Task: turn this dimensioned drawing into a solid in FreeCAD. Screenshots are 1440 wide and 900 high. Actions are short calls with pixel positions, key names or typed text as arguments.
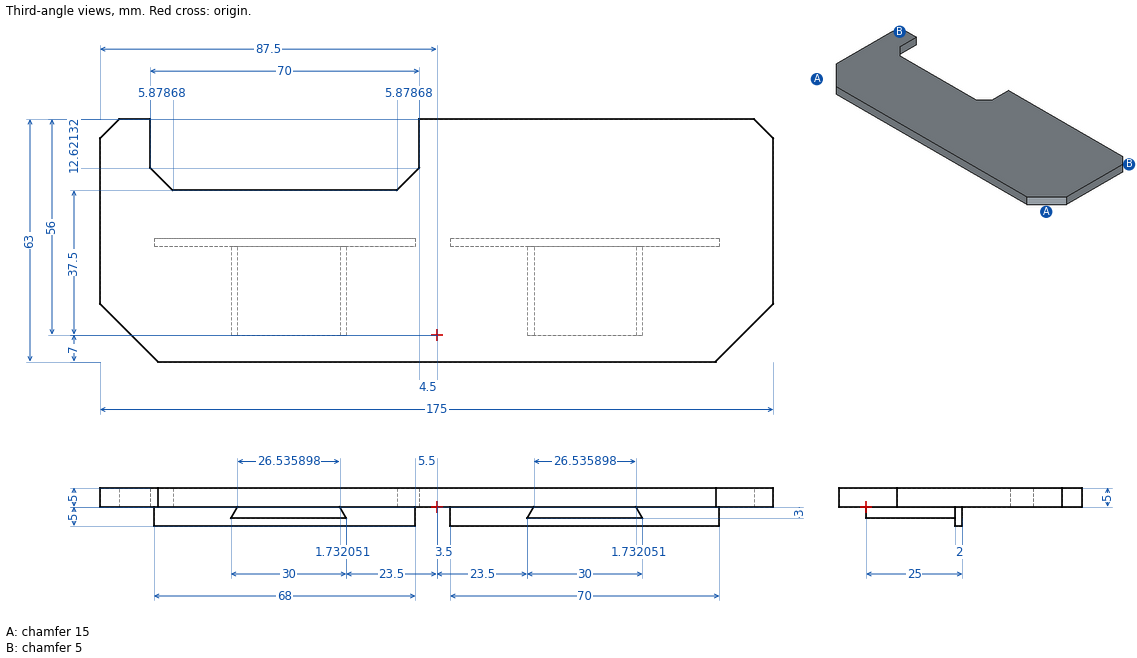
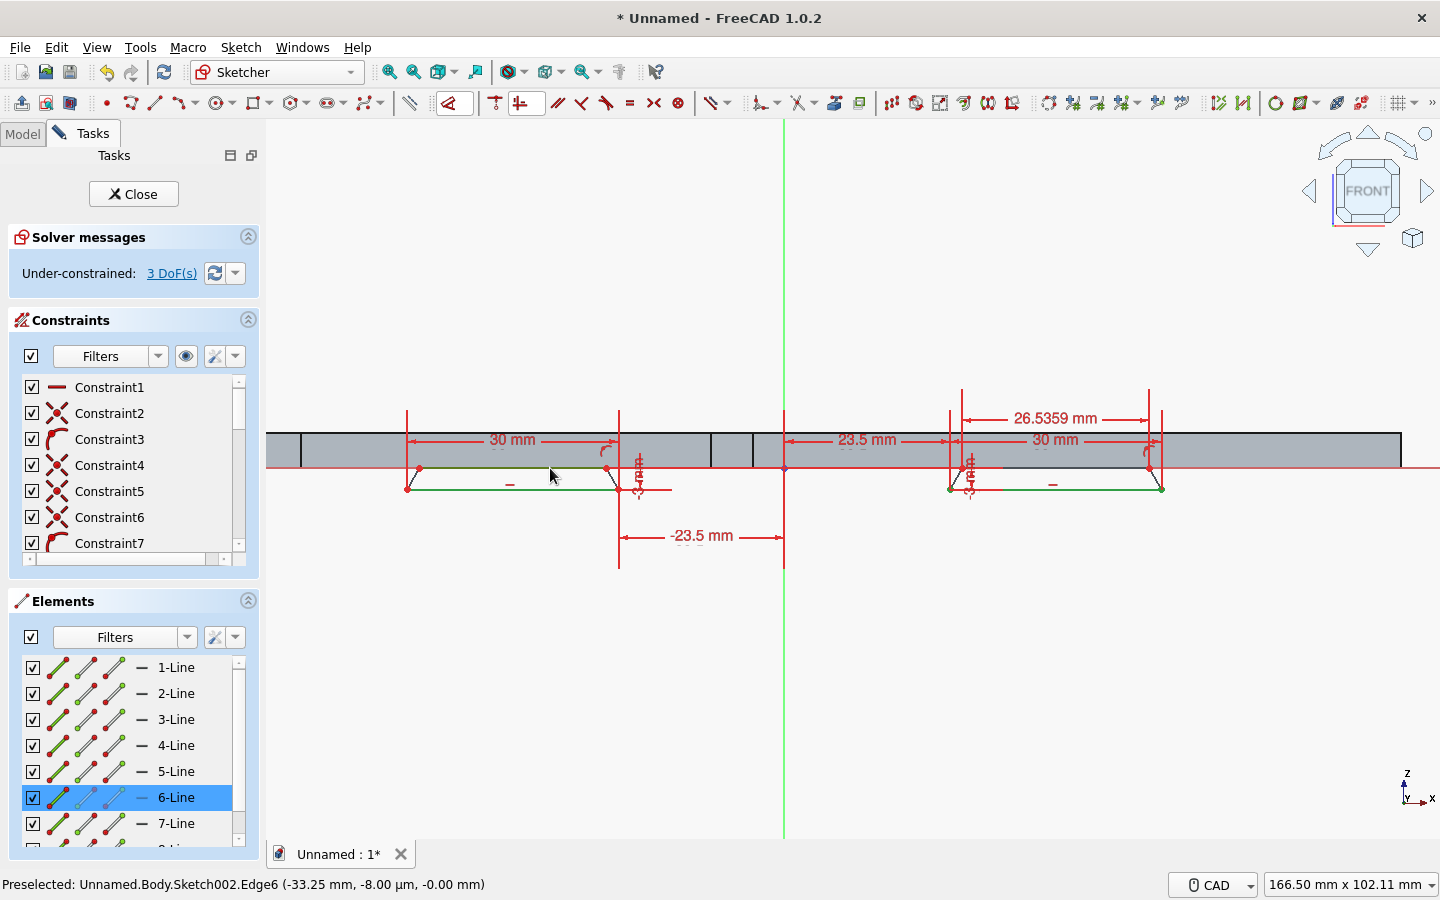
key(l)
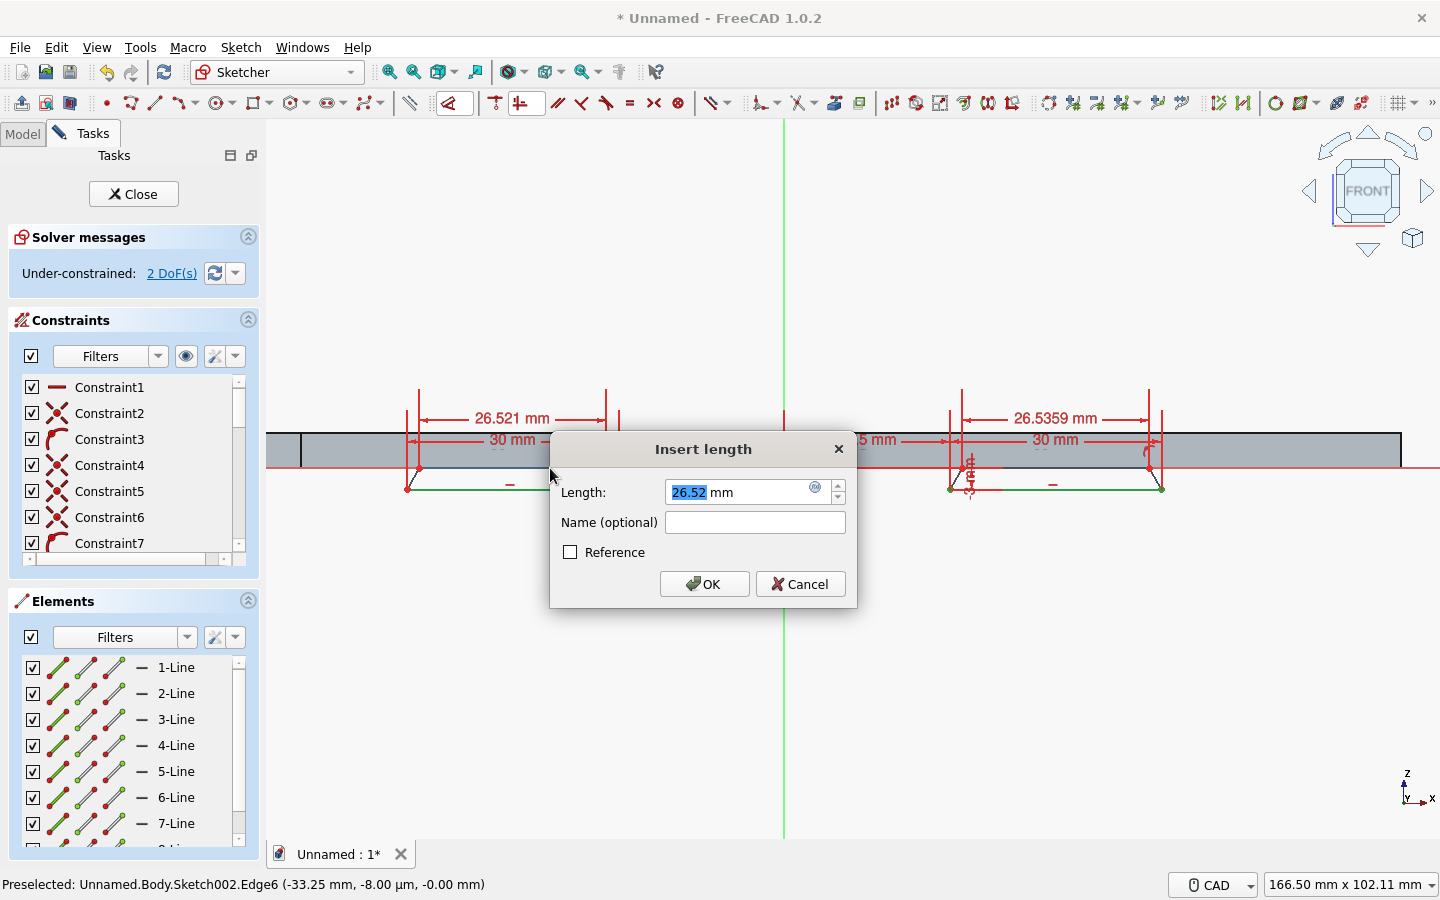
text(26.535898)
key(Return)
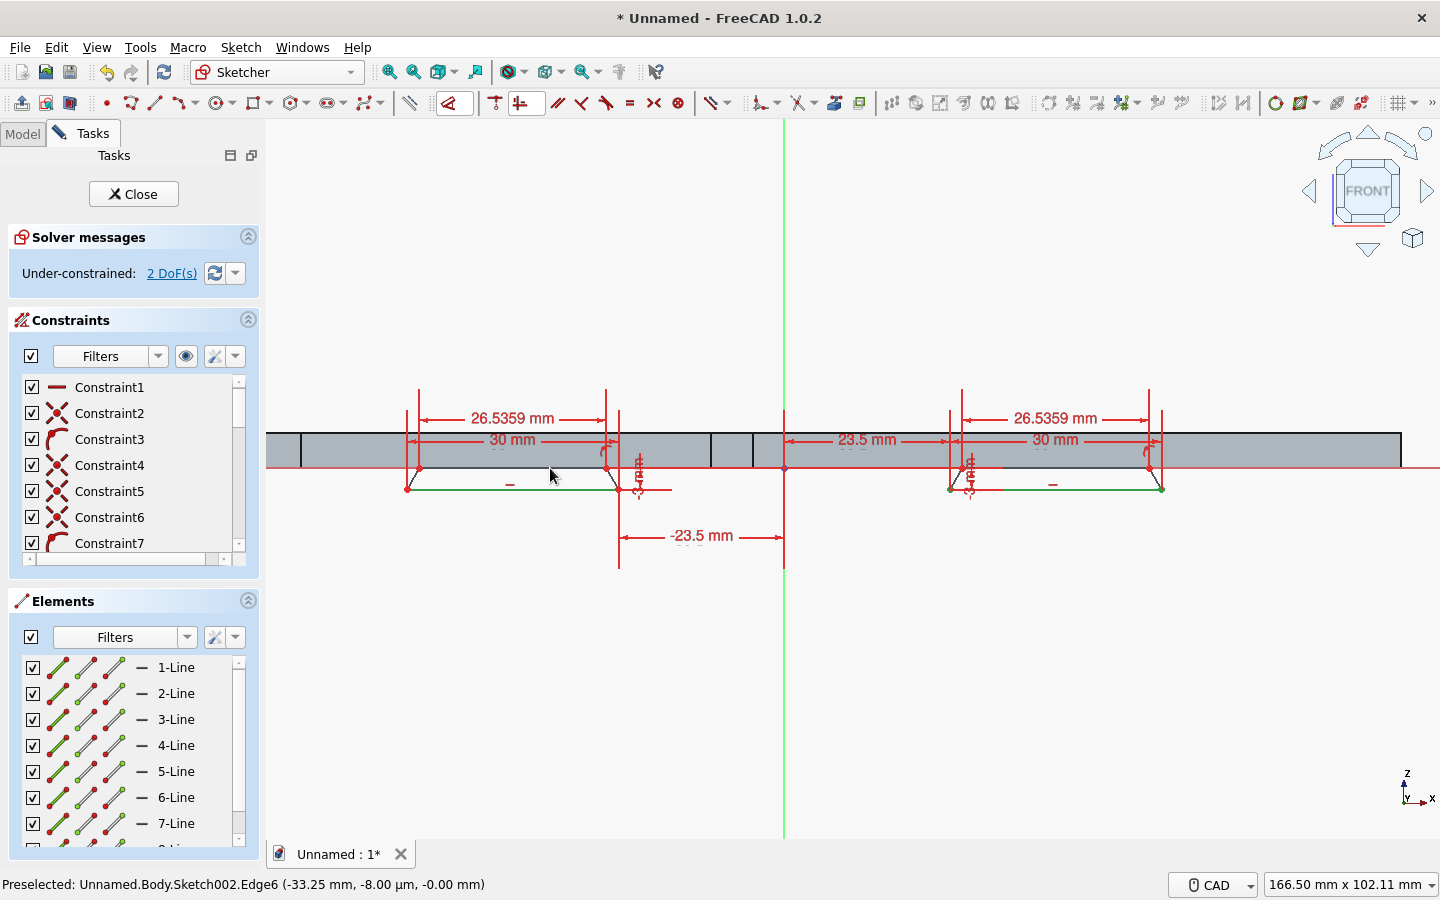
scroll(1155, 479, up, 6)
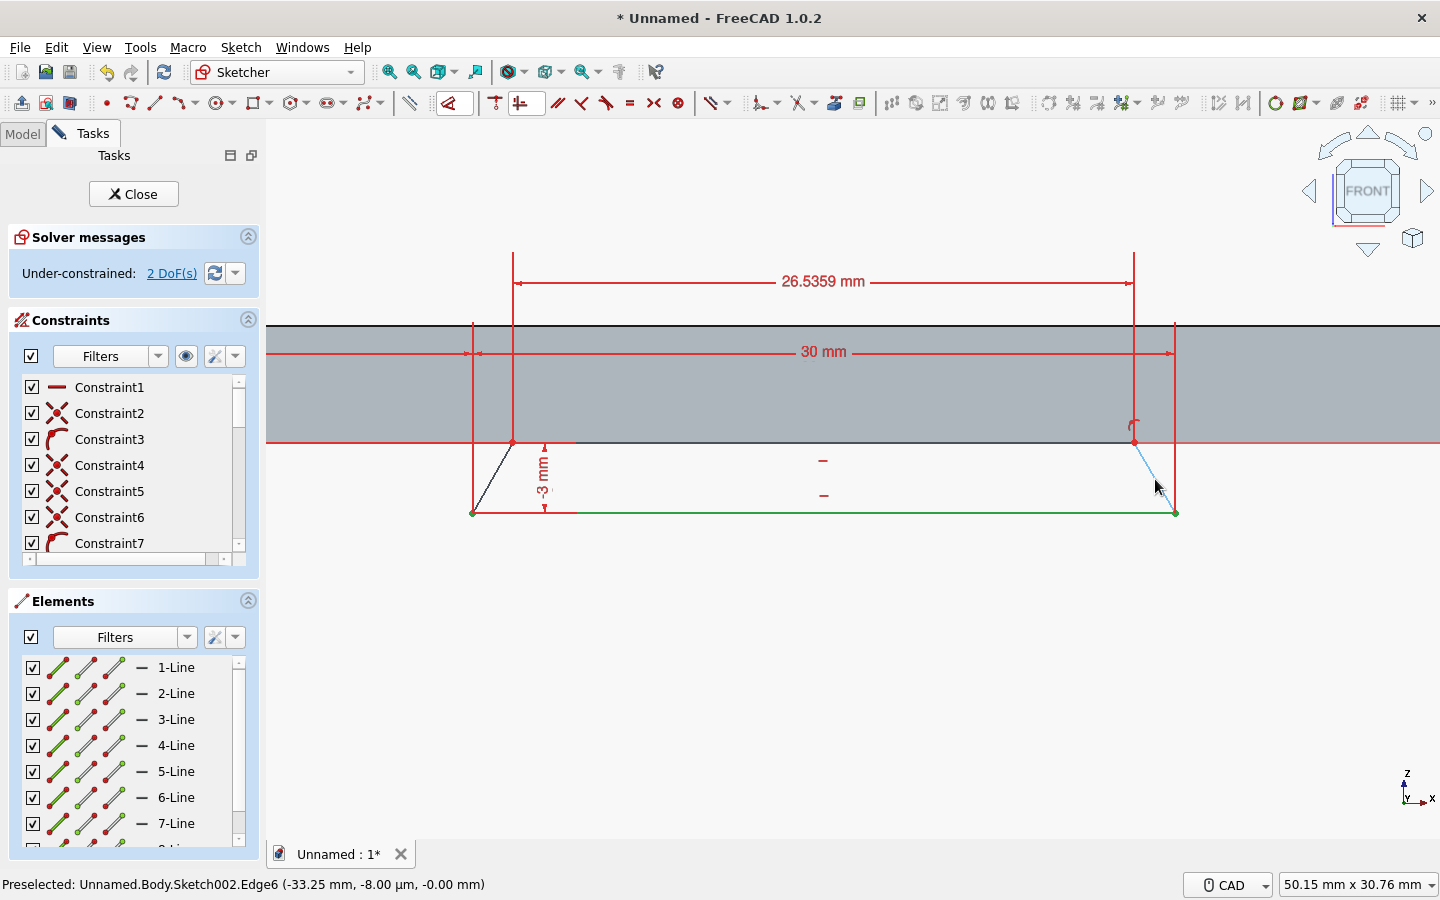
click(1155, 478)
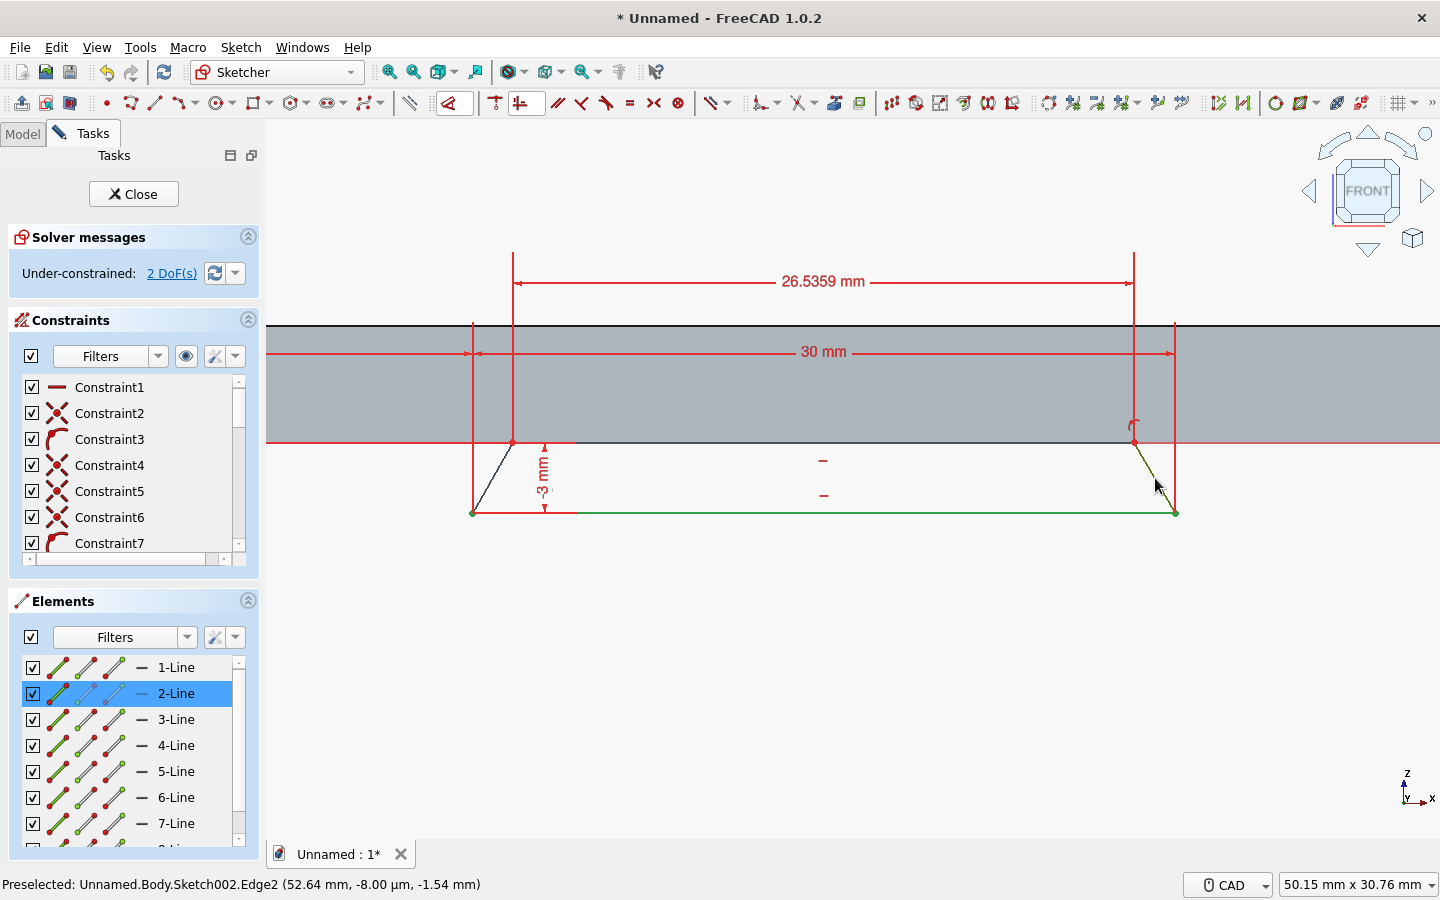
key(l)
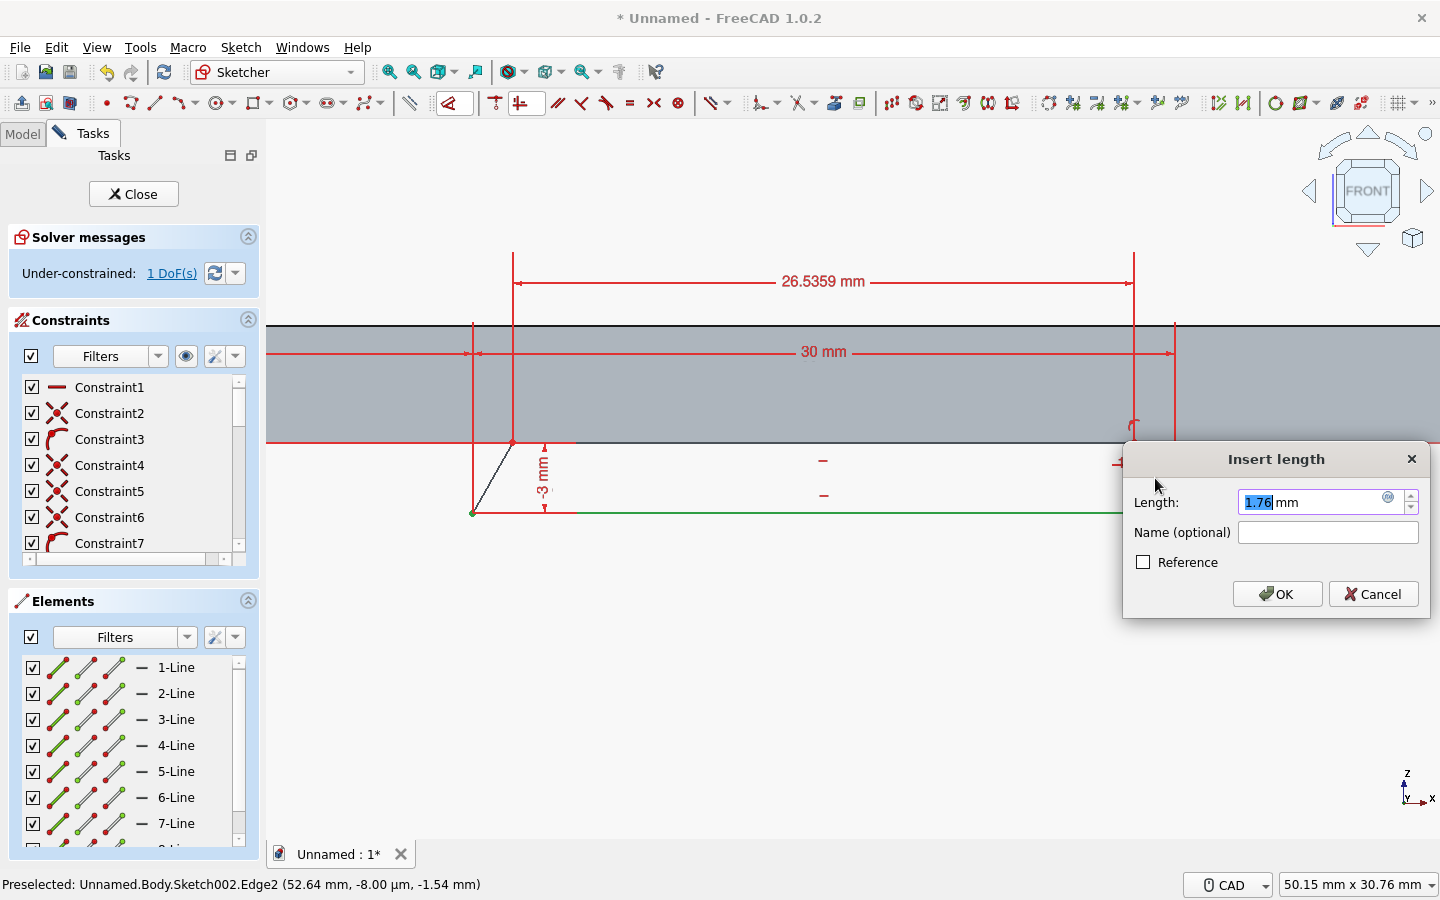
text(1.732051)
key(Return)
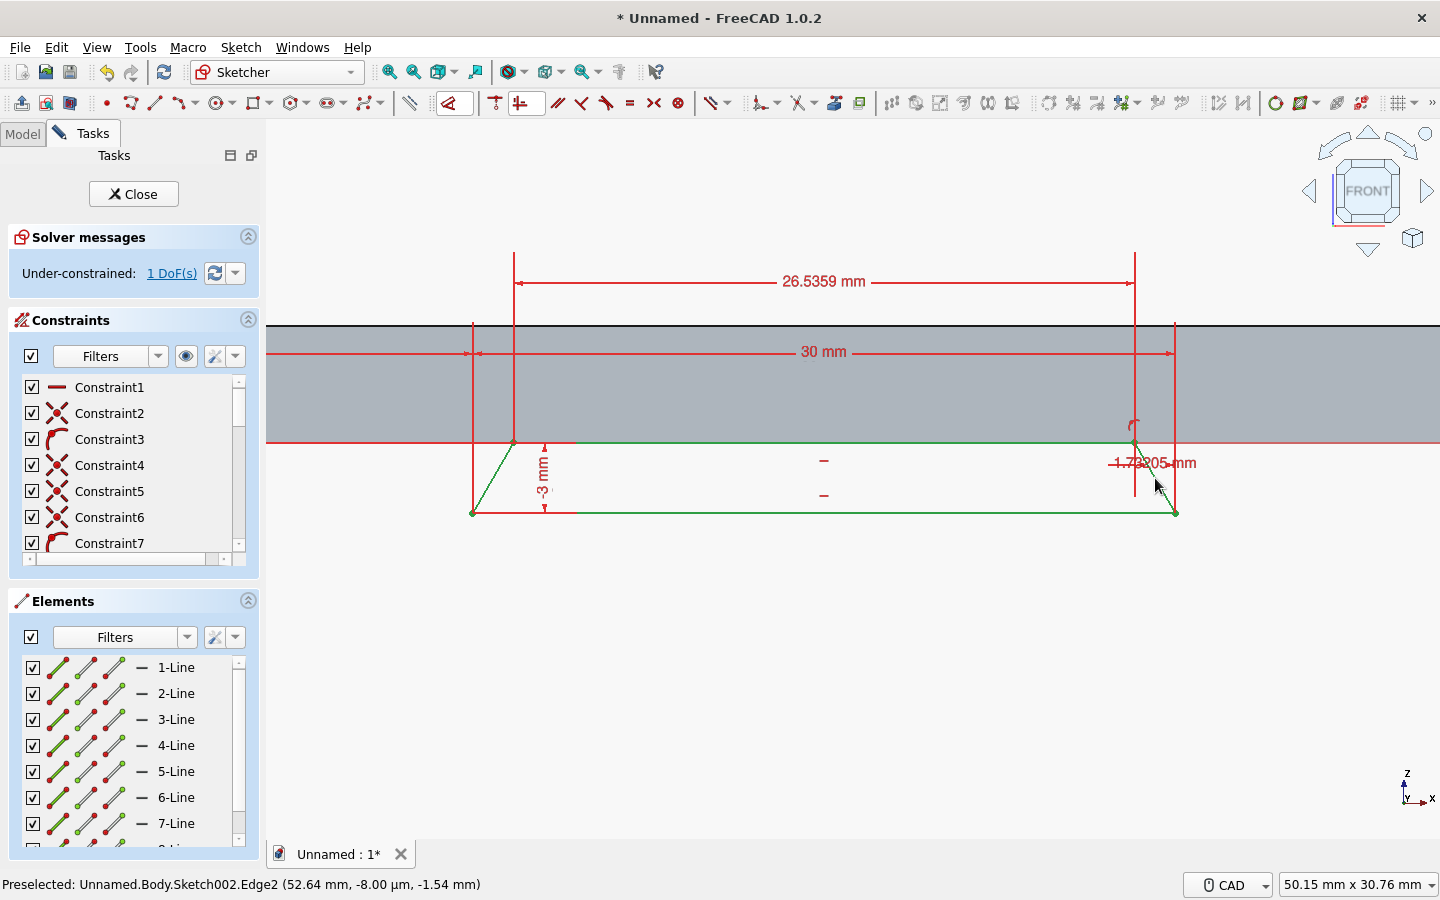
scroll(1156, 479, down, 6)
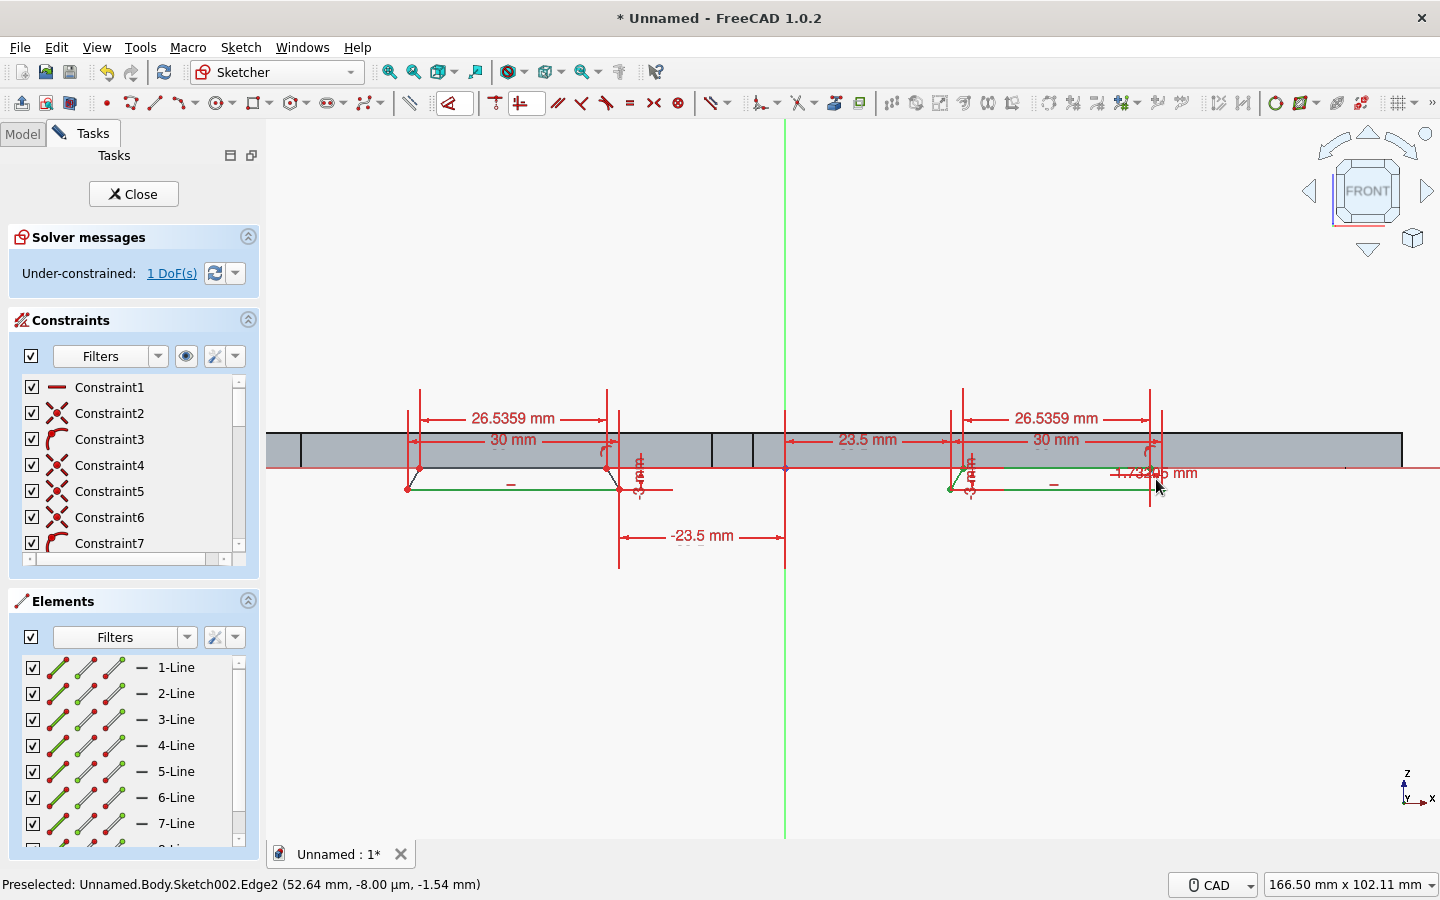
scroll(616, 483, up, 6)